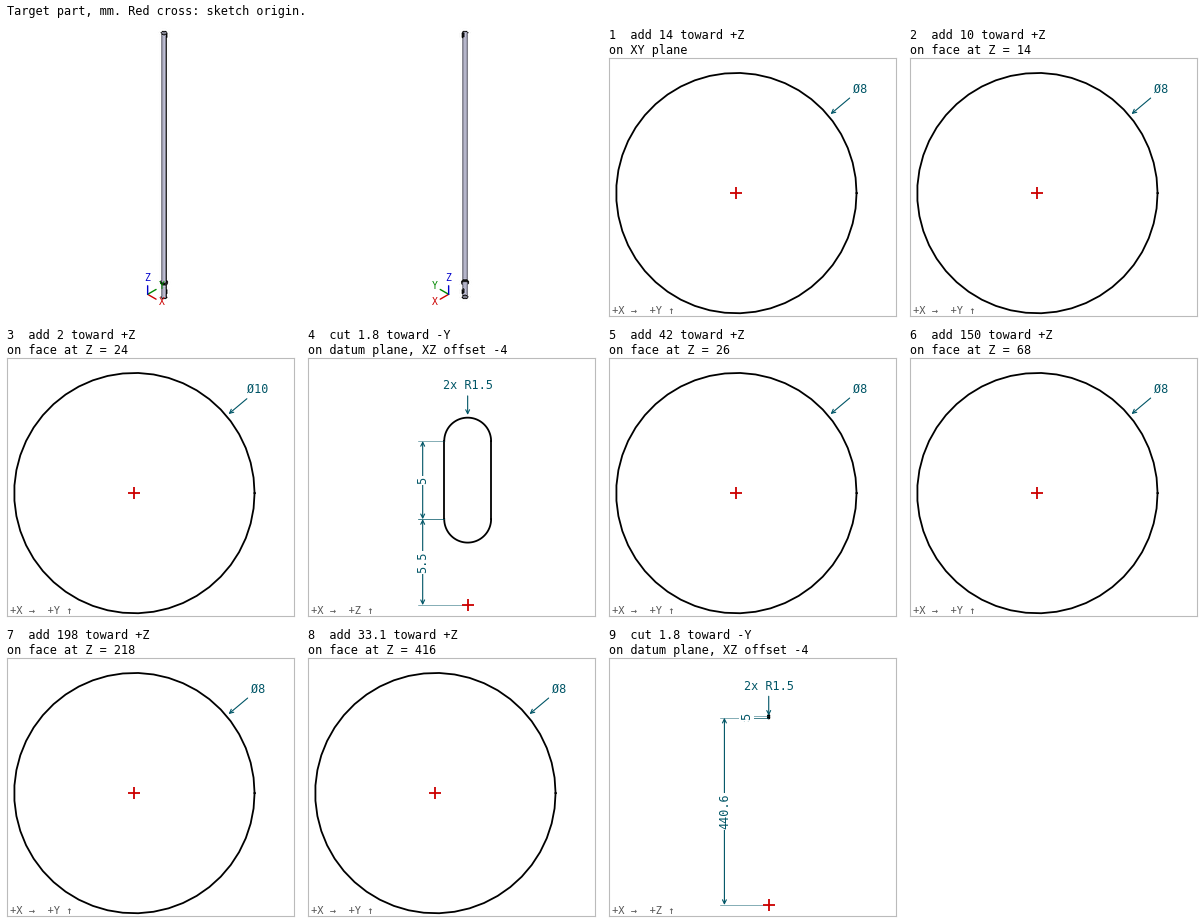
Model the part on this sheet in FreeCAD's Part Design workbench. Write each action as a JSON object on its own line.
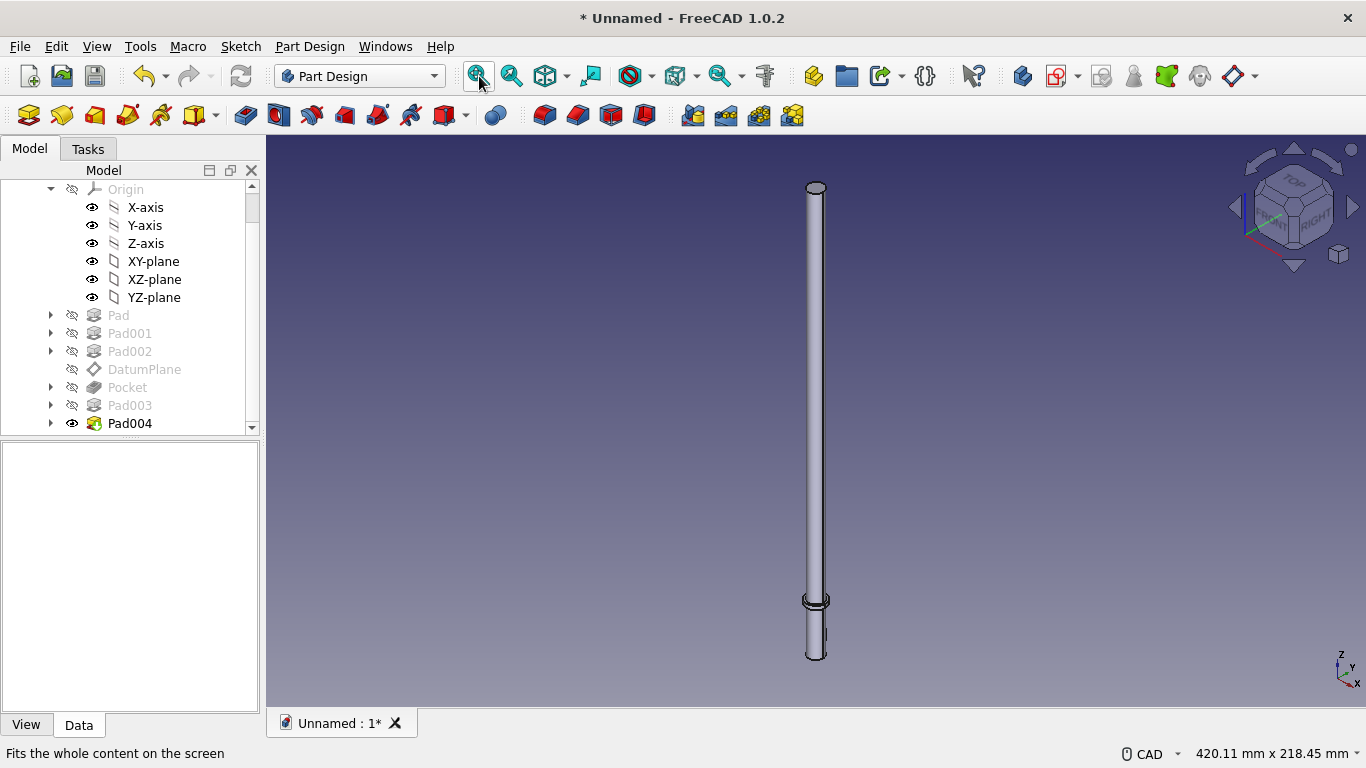
{"action": "key", "text": "2"}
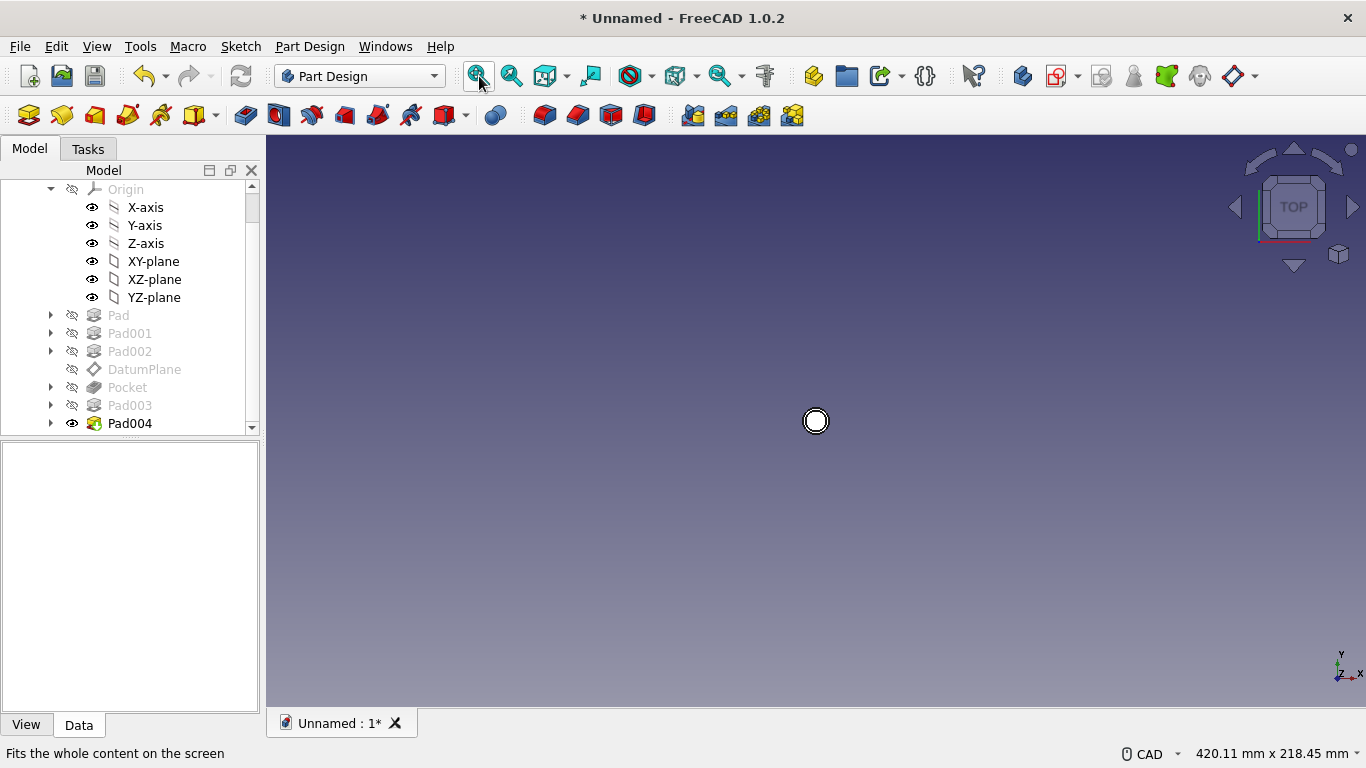
{"action": "left_click", "coordinate": [479, 76]}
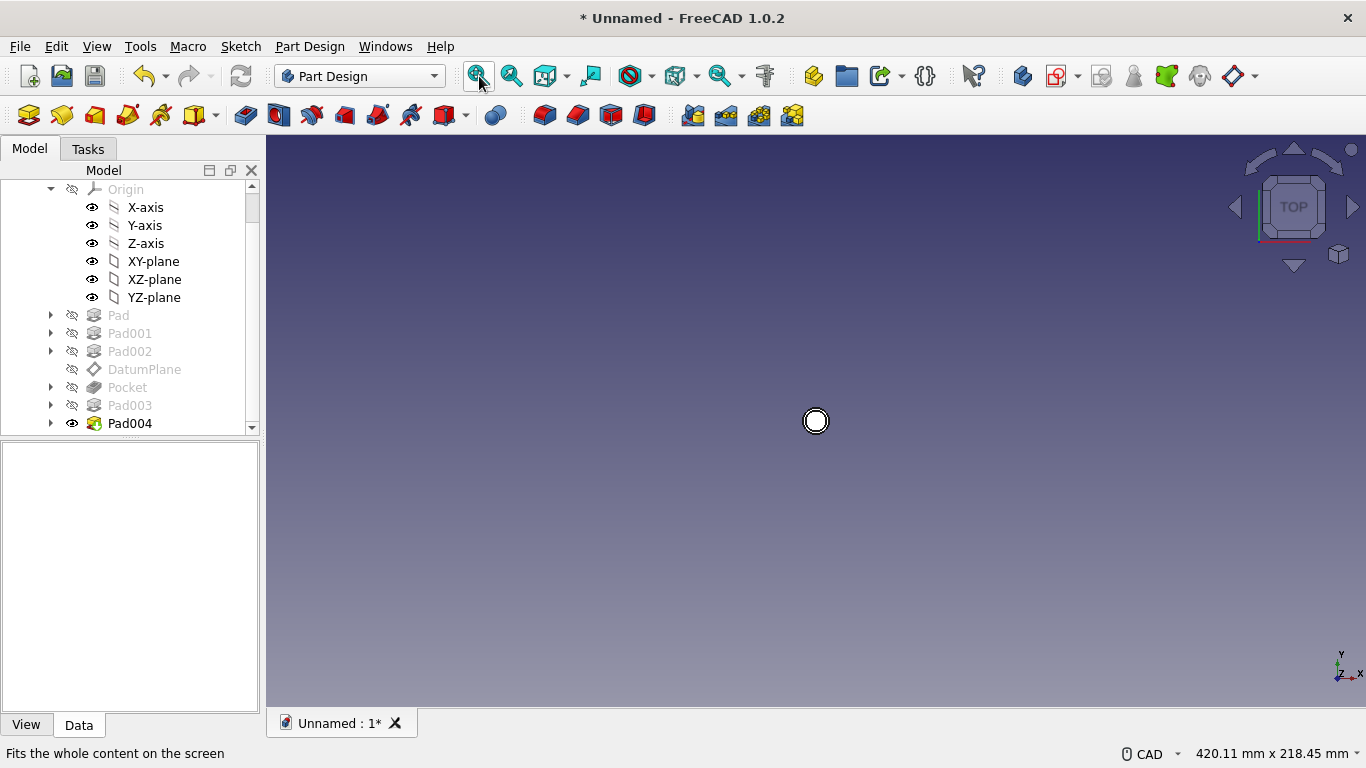
{"action": "left_click", "coordinate": [816, 420]}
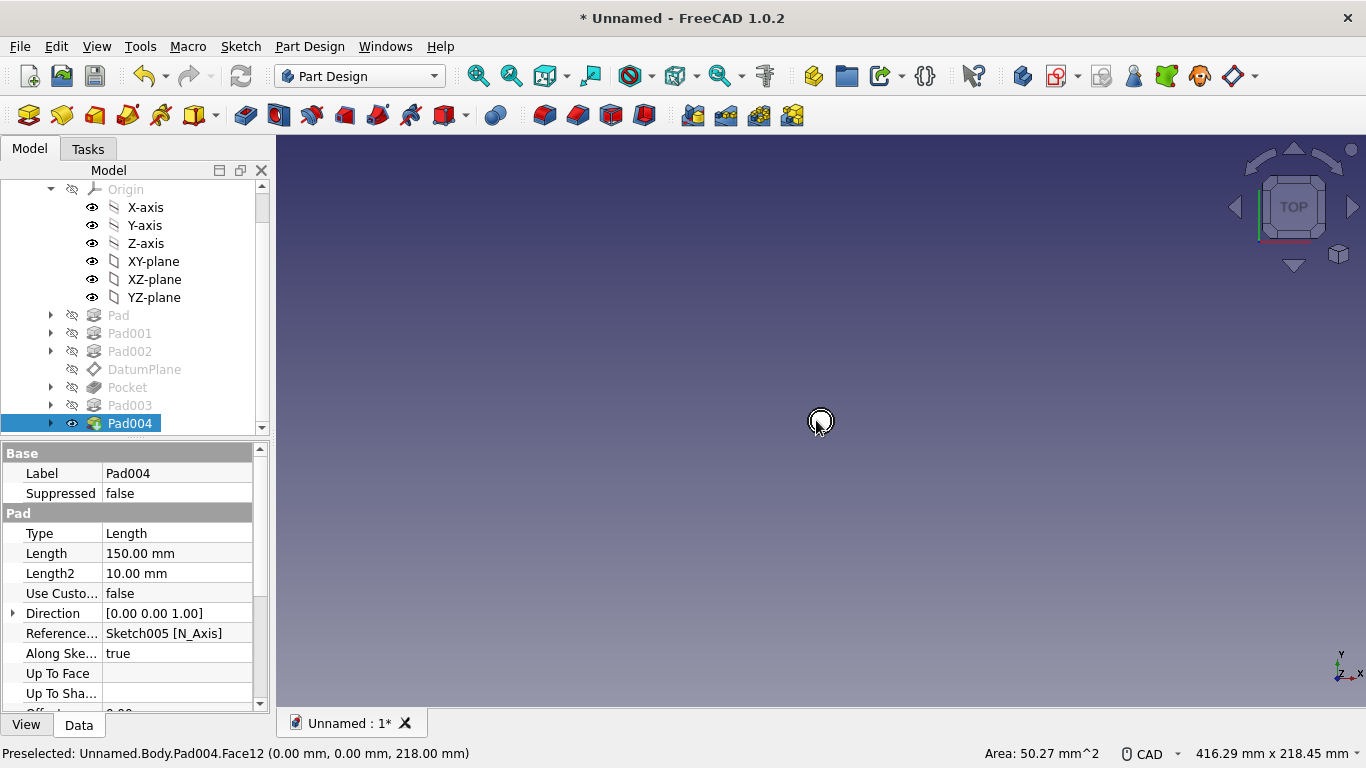
{"action": "left_click", "coordinate": [1056, 76]}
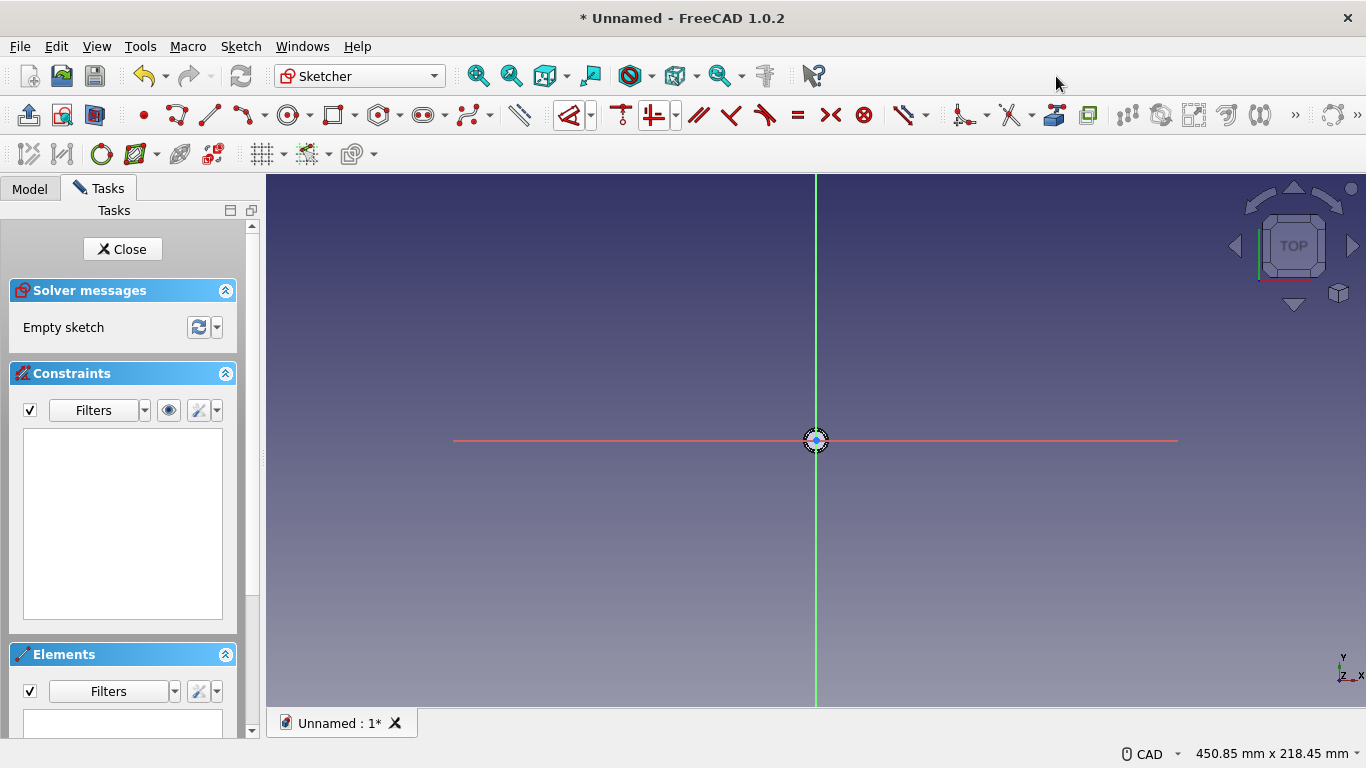
{"action": "scroll", "coordinate": [820, 440], "scroll_direction": "up", "scroll_amount": 14}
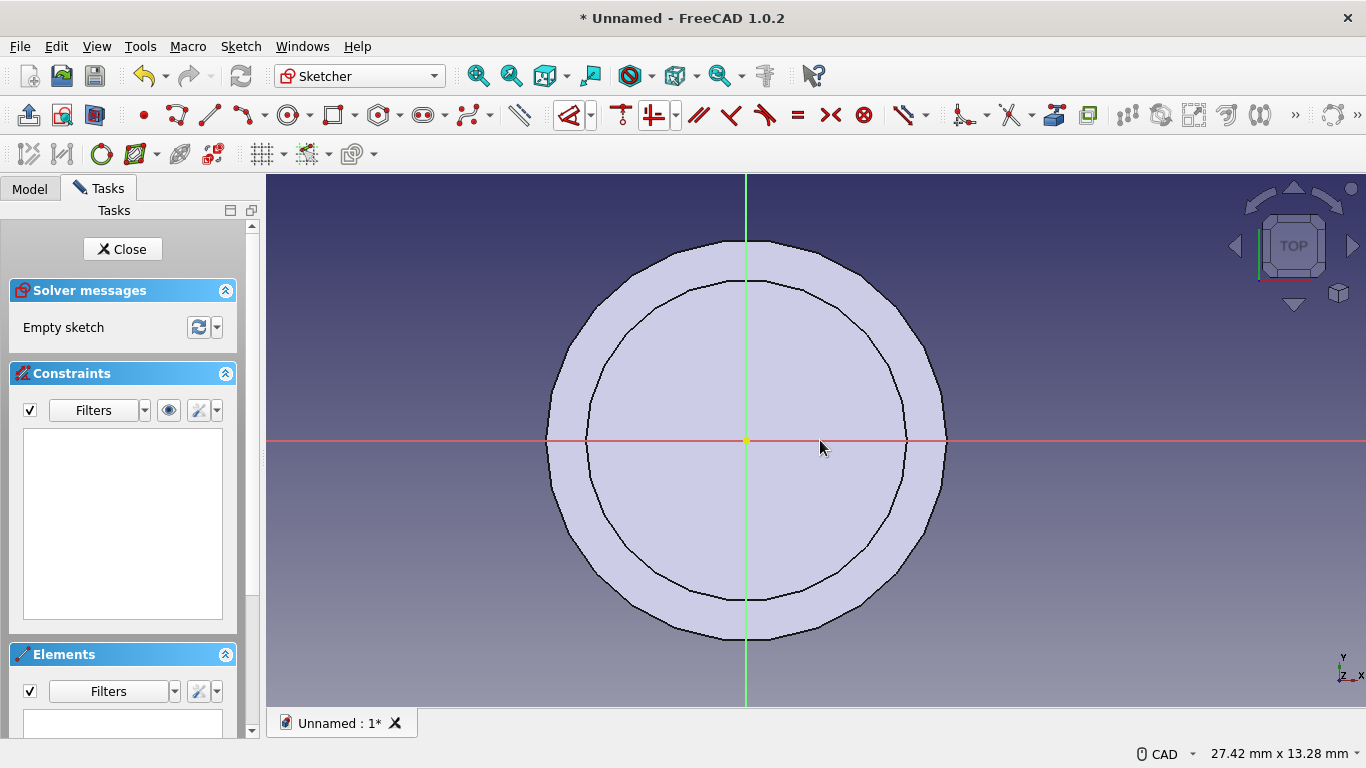
{"action": "left_click", "coordinate": [288, 116]}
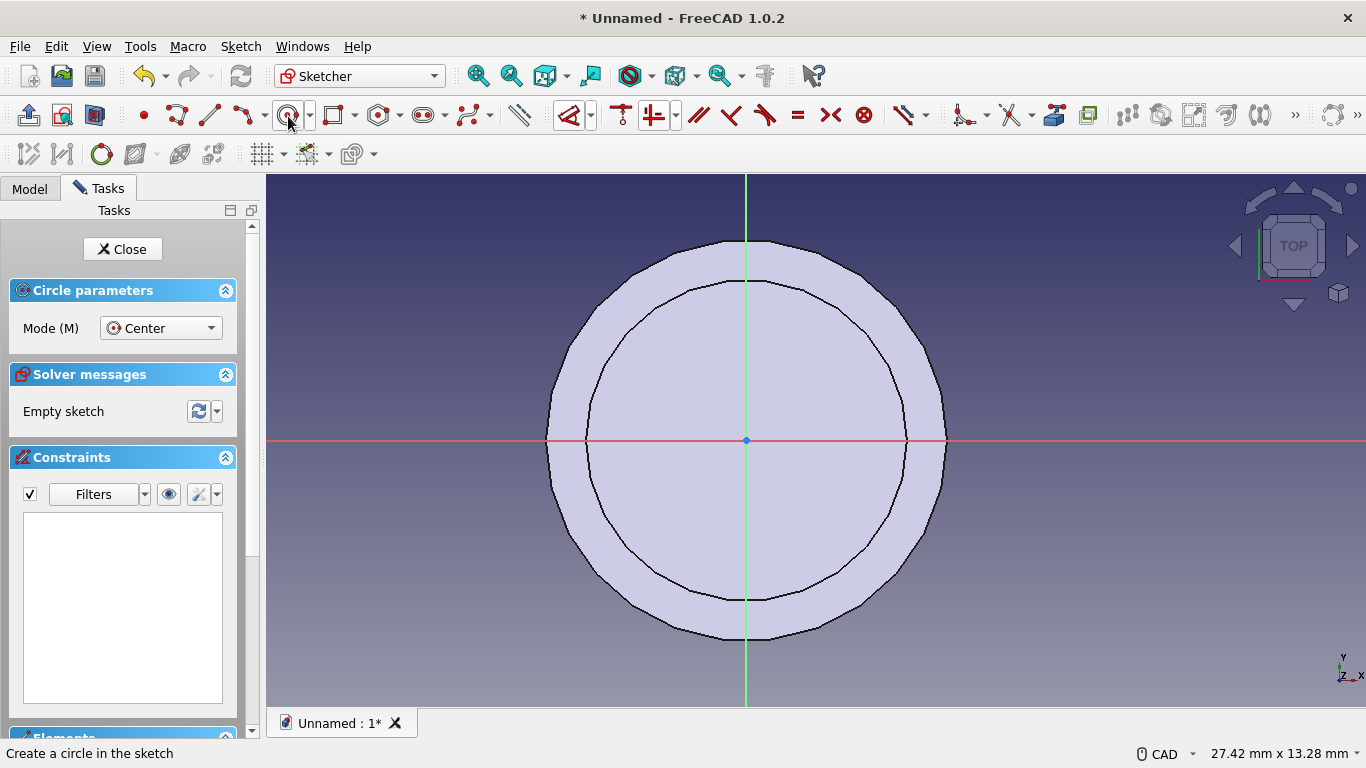
{"action": "left_click", "coordinate": [746, 440]}
{"action": "left_click", "coordinate": [860, 327]}
{"action": "key", "text": "Escape"}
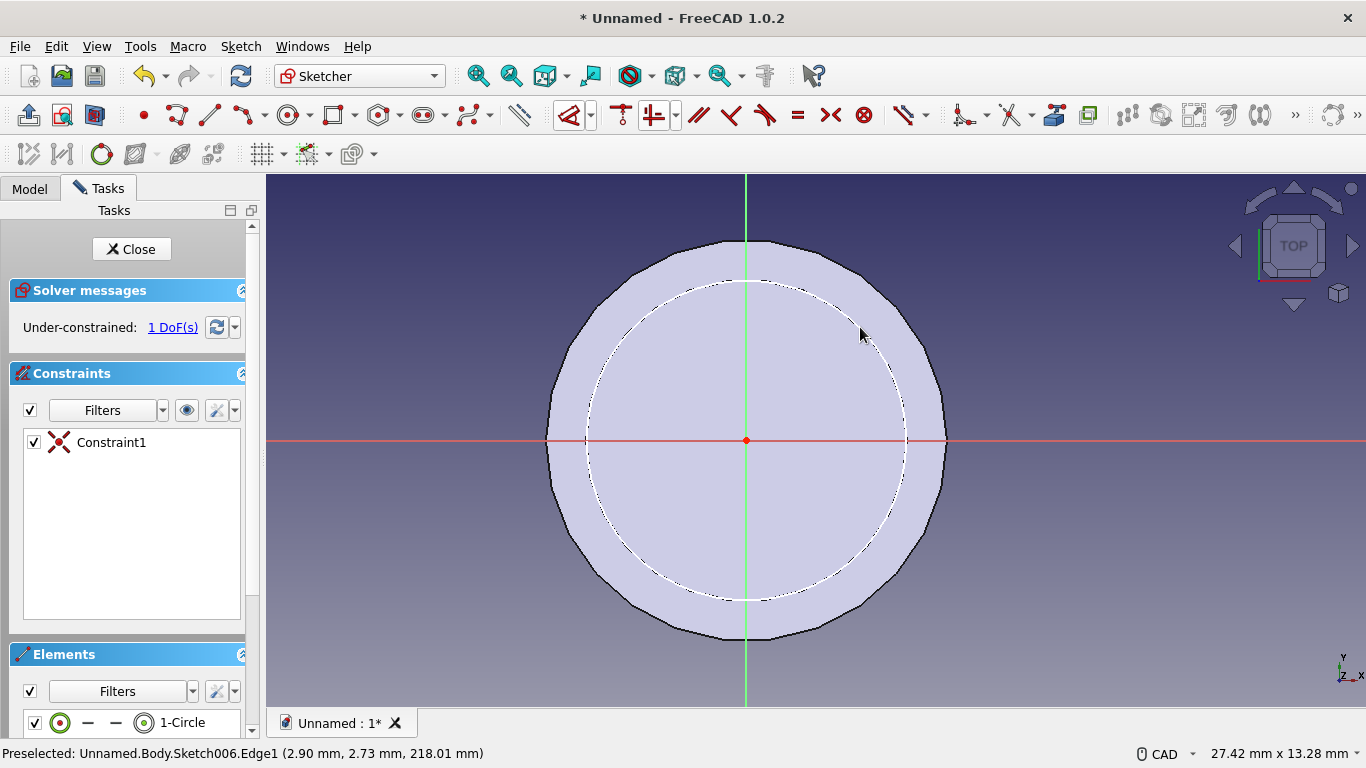
{"action": "left_click", "coordinate": [859, 327]}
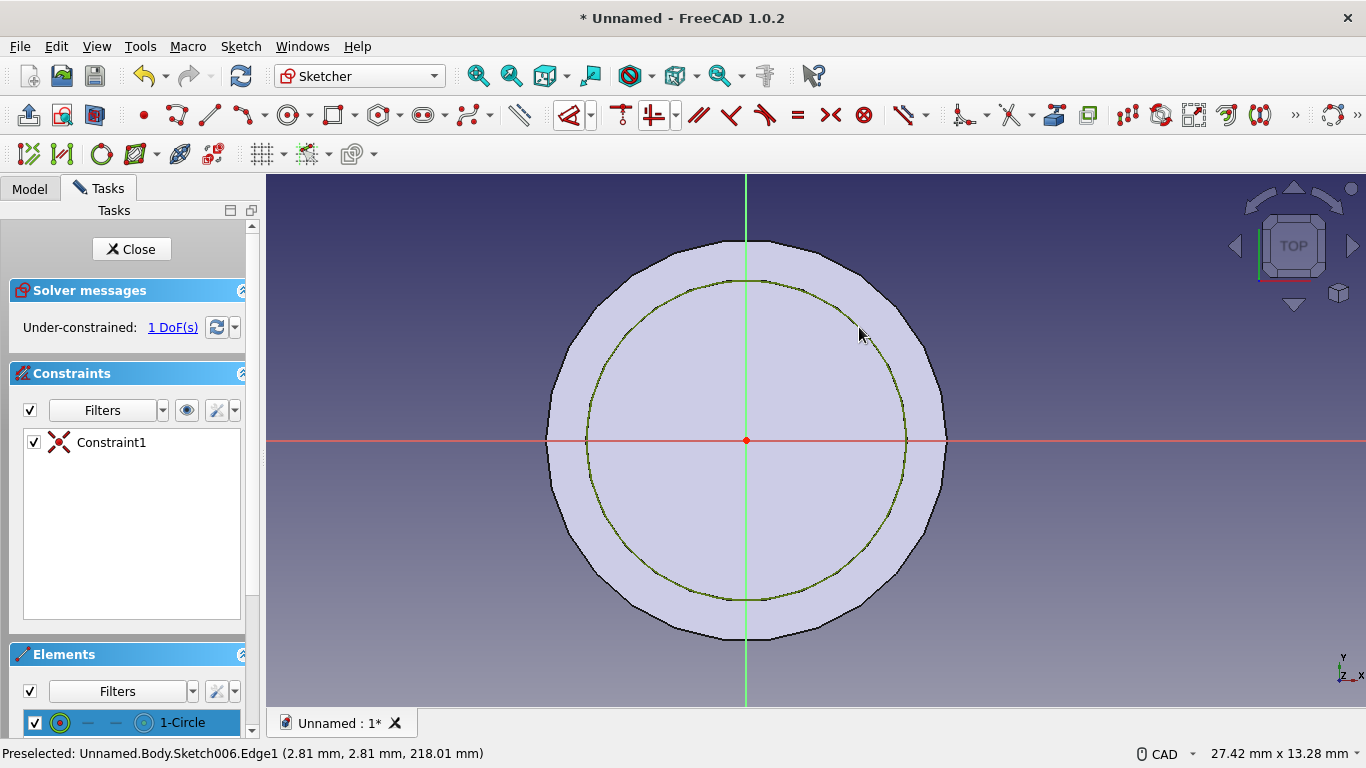
{"action": "key", "text": "k o"}